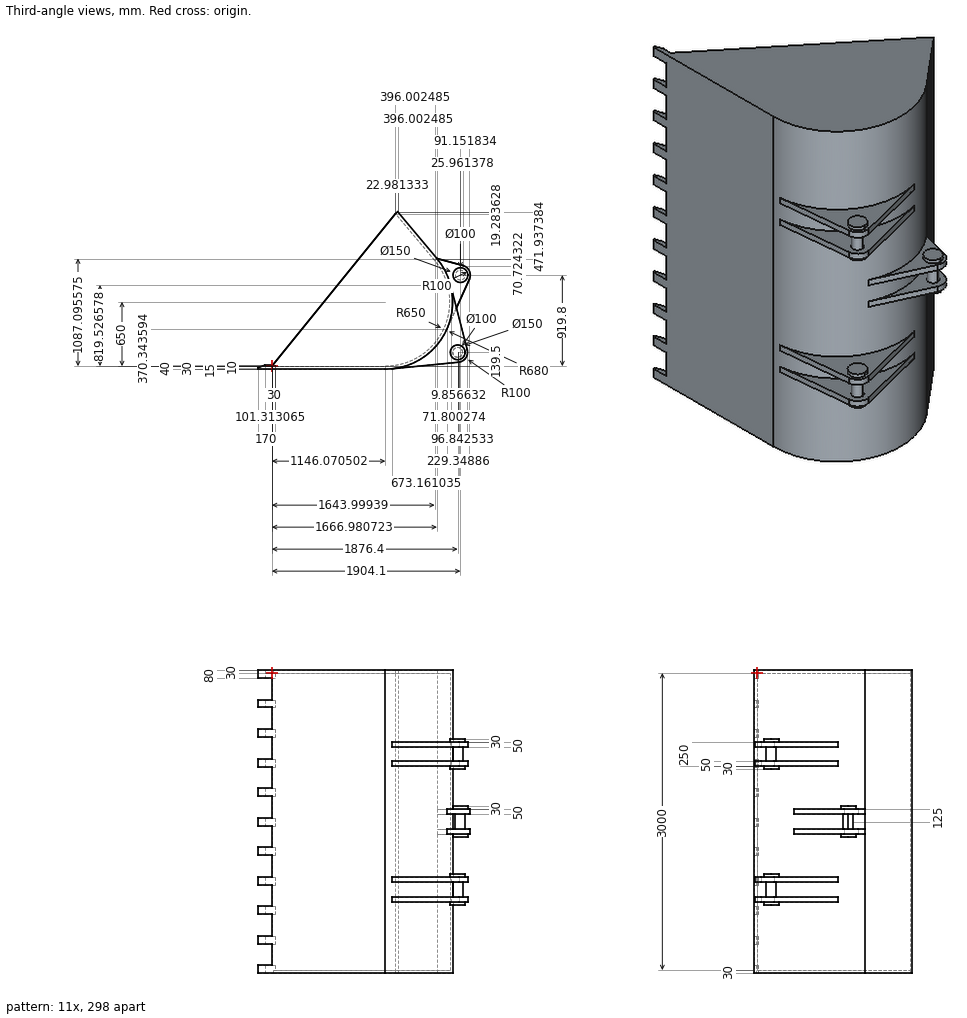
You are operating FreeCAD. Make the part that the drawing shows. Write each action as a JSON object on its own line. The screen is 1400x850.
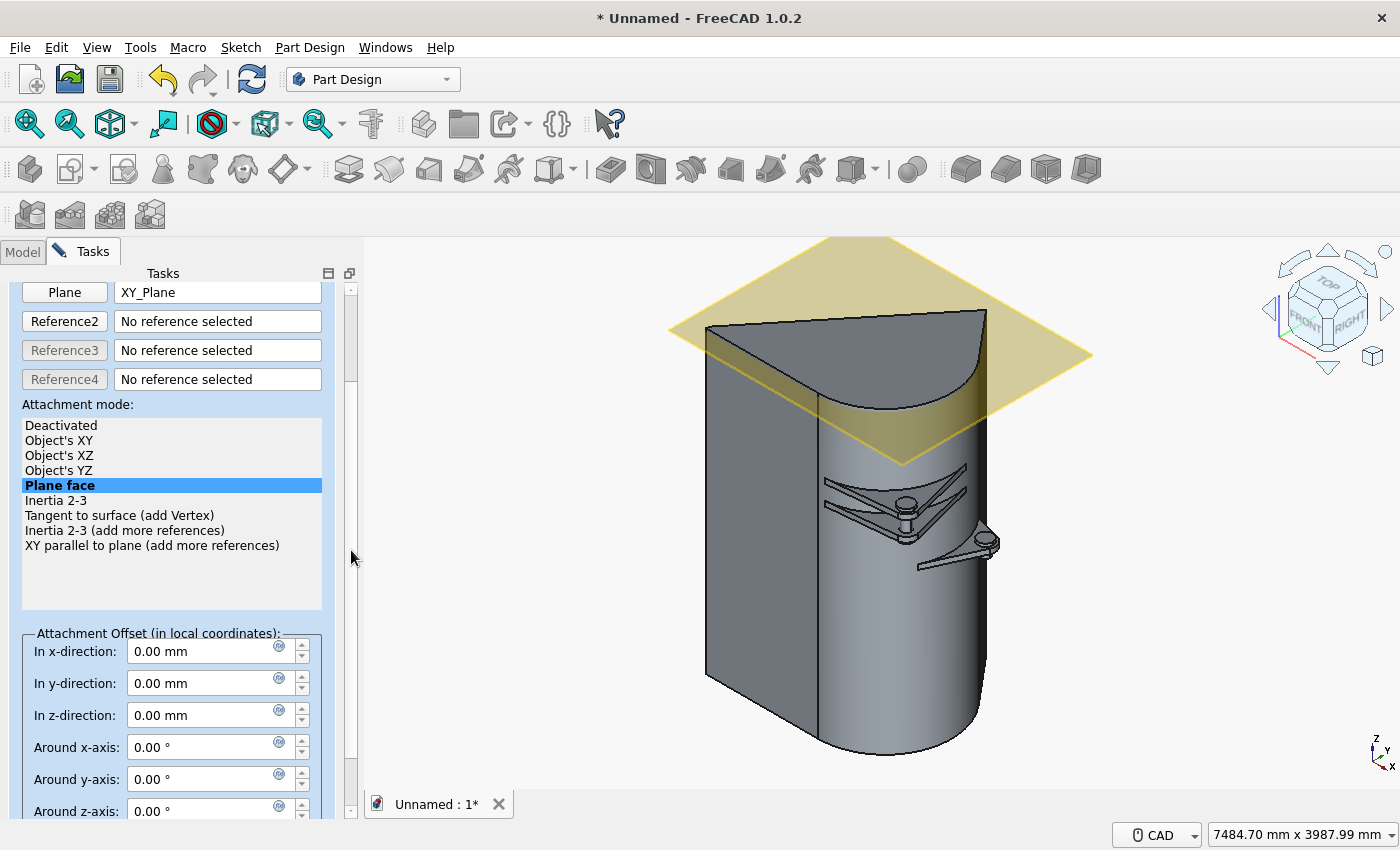
{"action": "triple_click", "coordinate": [210, 715]}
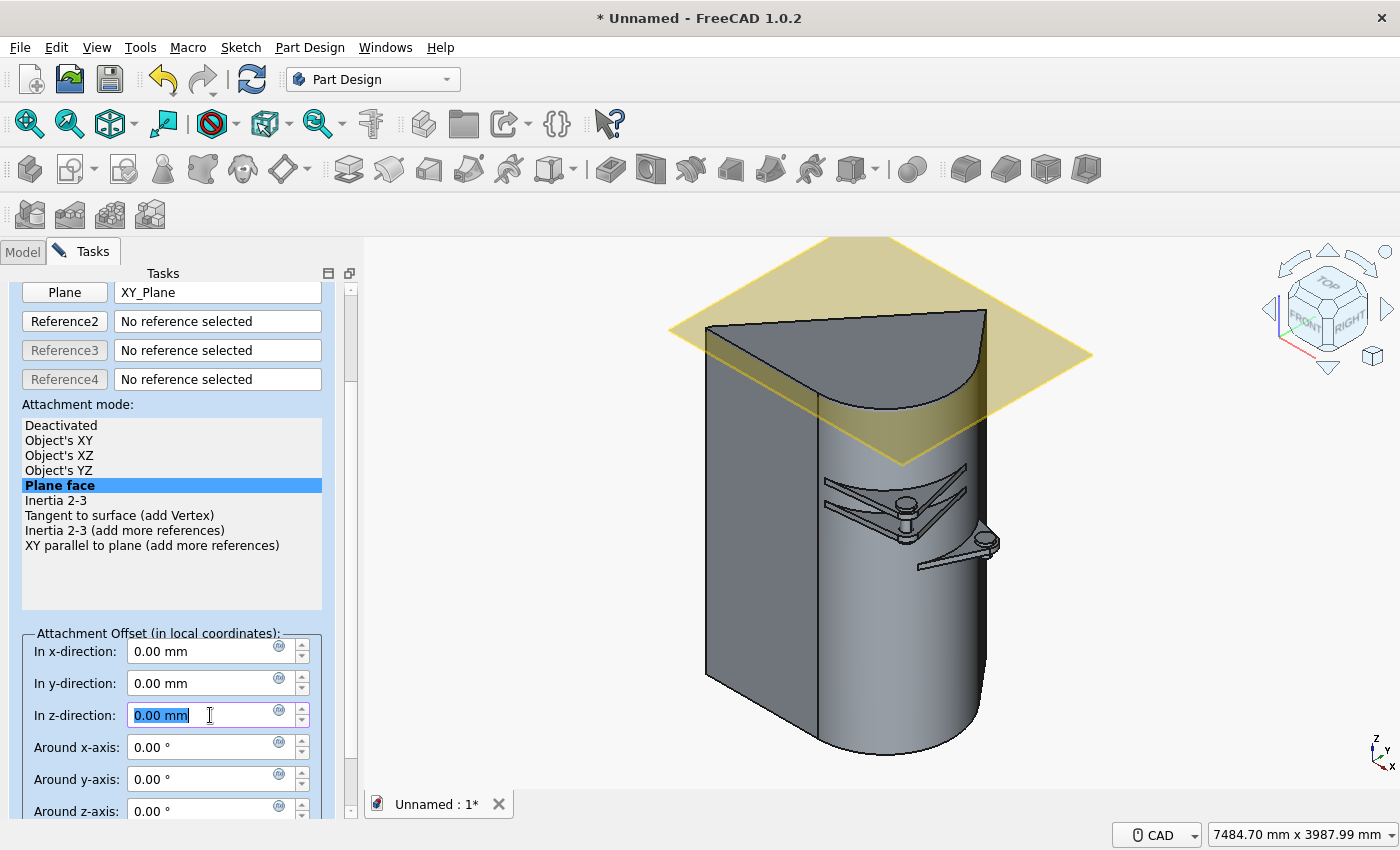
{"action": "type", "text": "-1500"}
{"action": "key", "text": "Tab"}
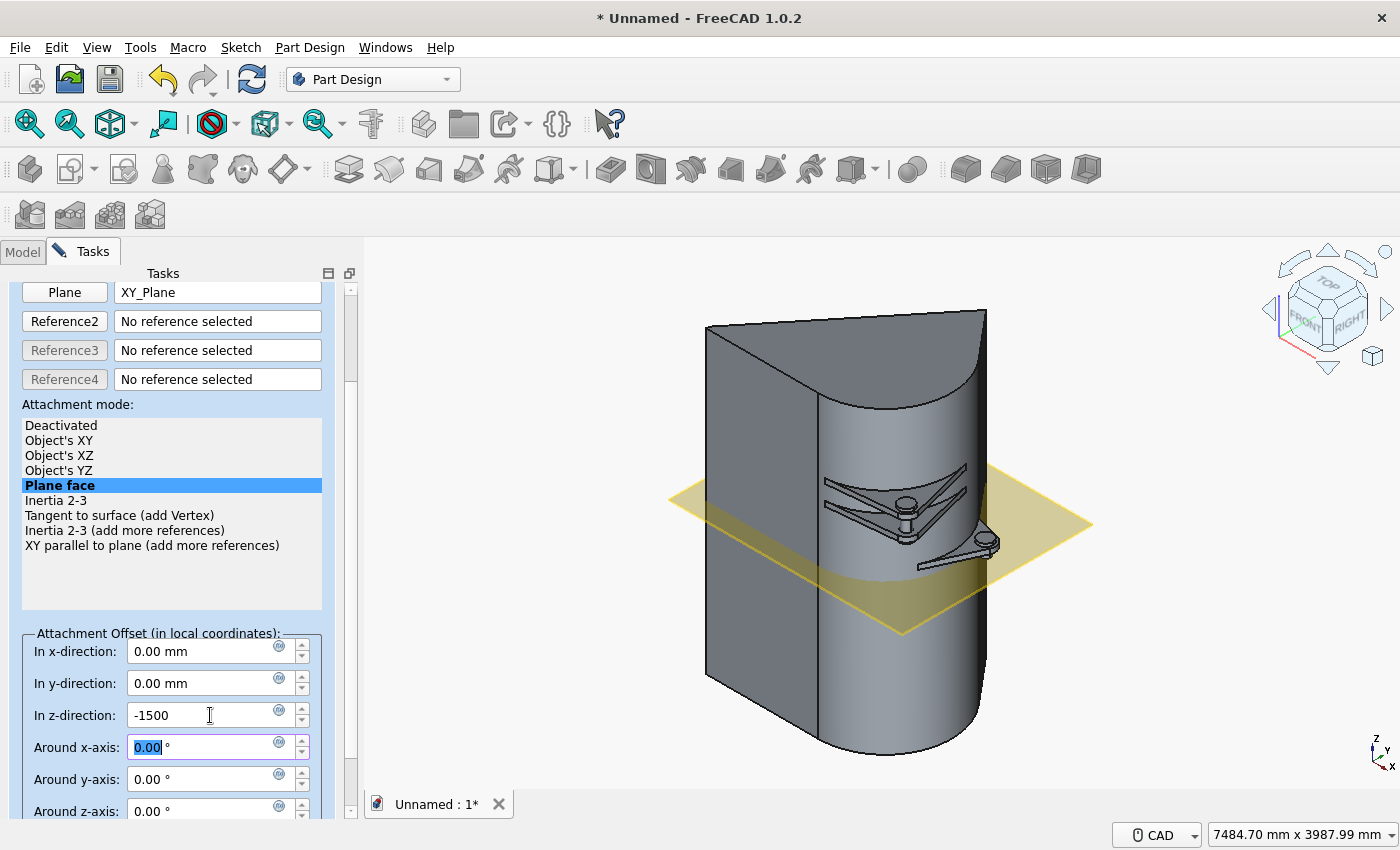
{"action": "scroll", "coordinate": [351, 550], "scroll_direction": "up", "scroll_amount": 3}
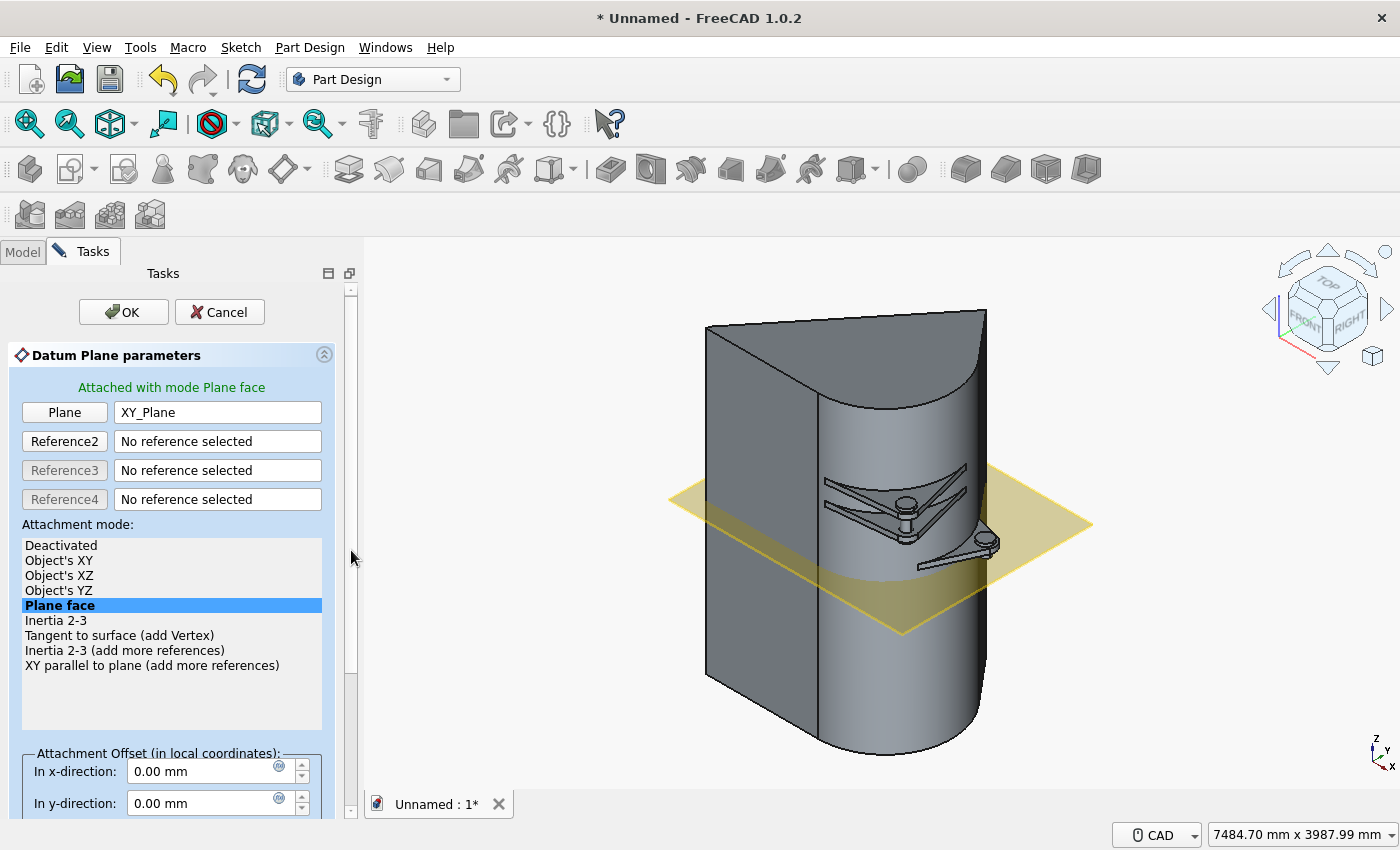
{"action": "left_click", "coordinate": [124, 312]}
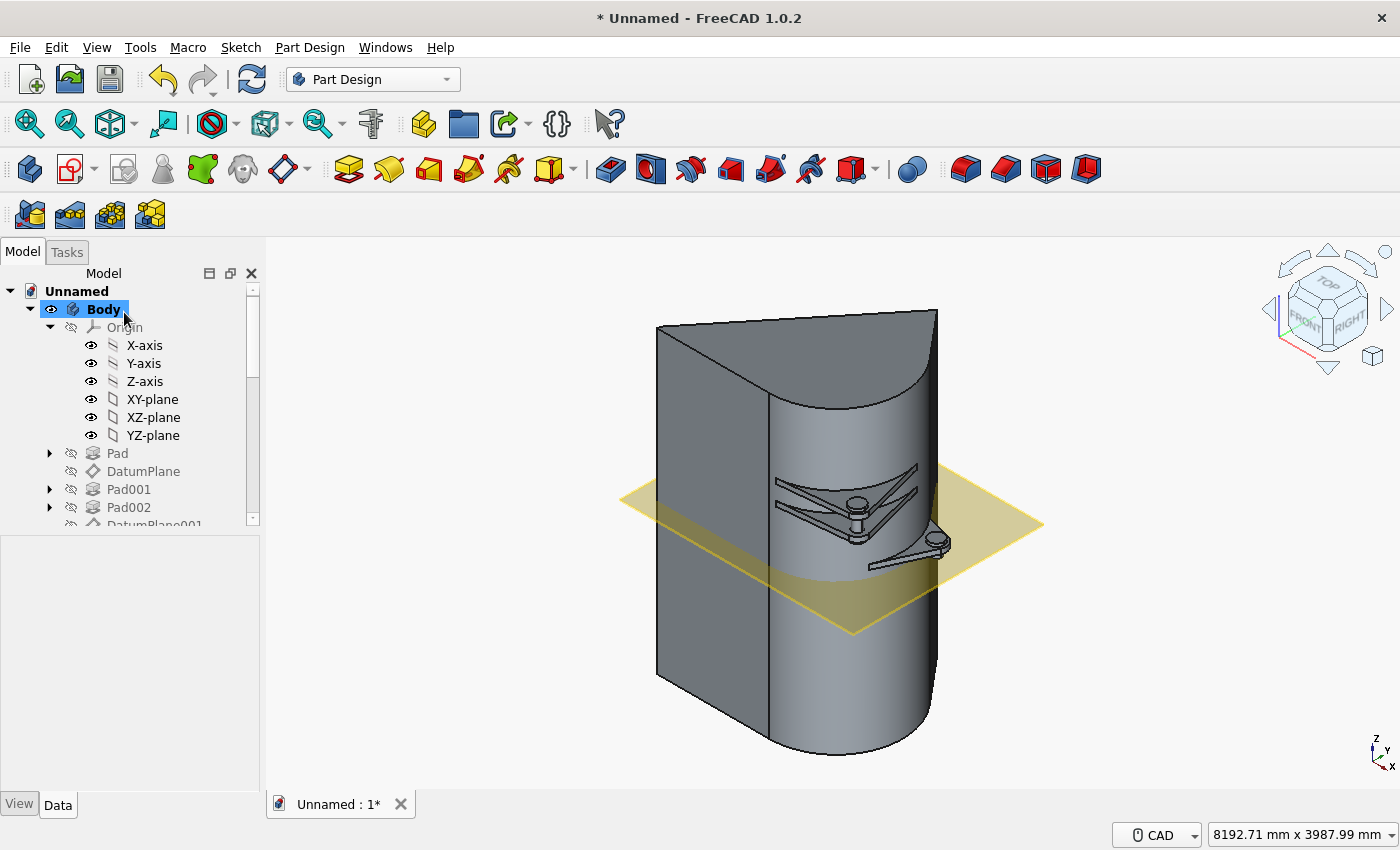
{"action": "scroll", "coordinate": [100, 413], "scroll_direction": "down", "scroll_amount": 3}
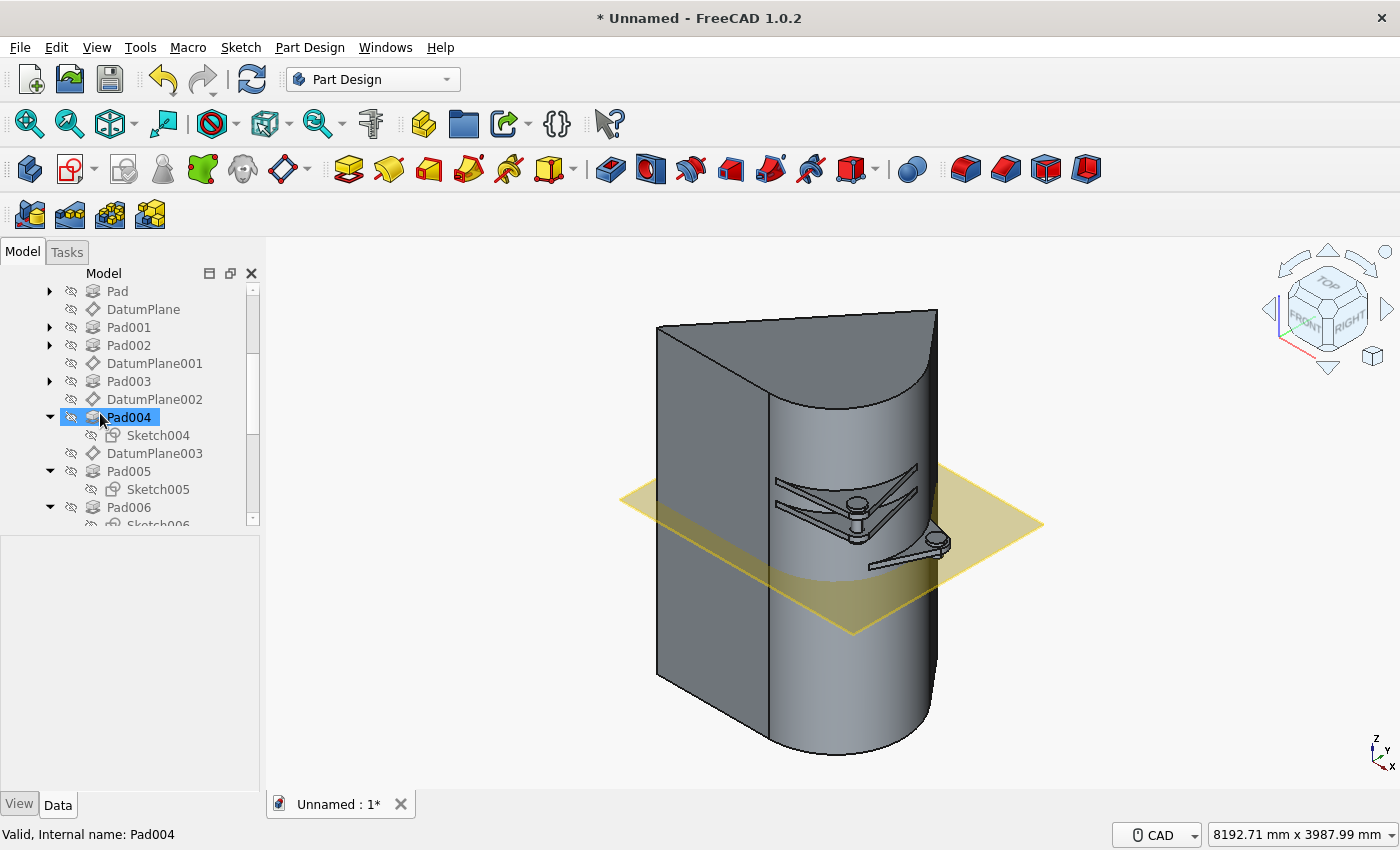
{"action": "left_click", "coordinate": [116, 381]}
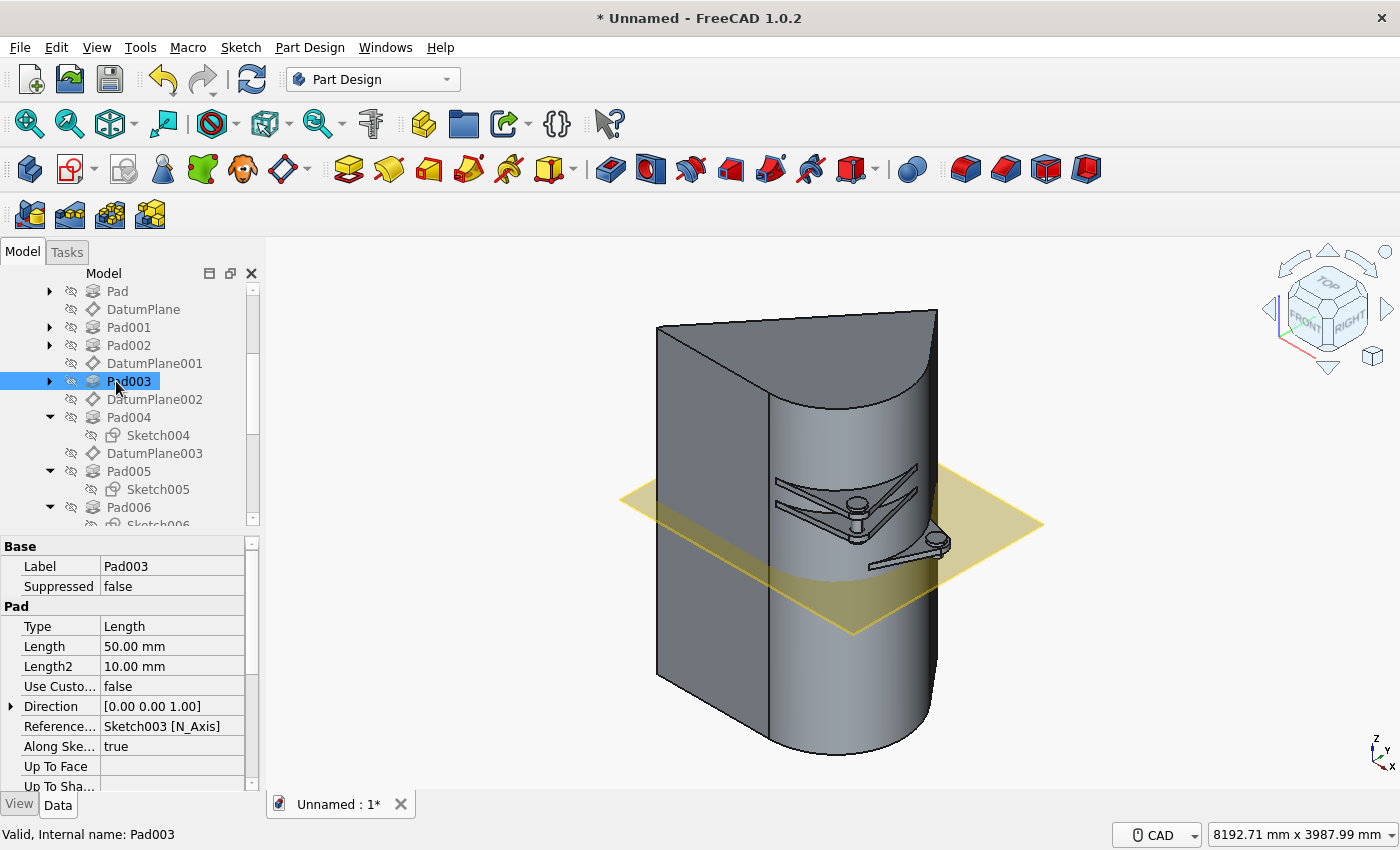
{"action": "left_click", "coordinate": [116, 417], "text": "ctrl"}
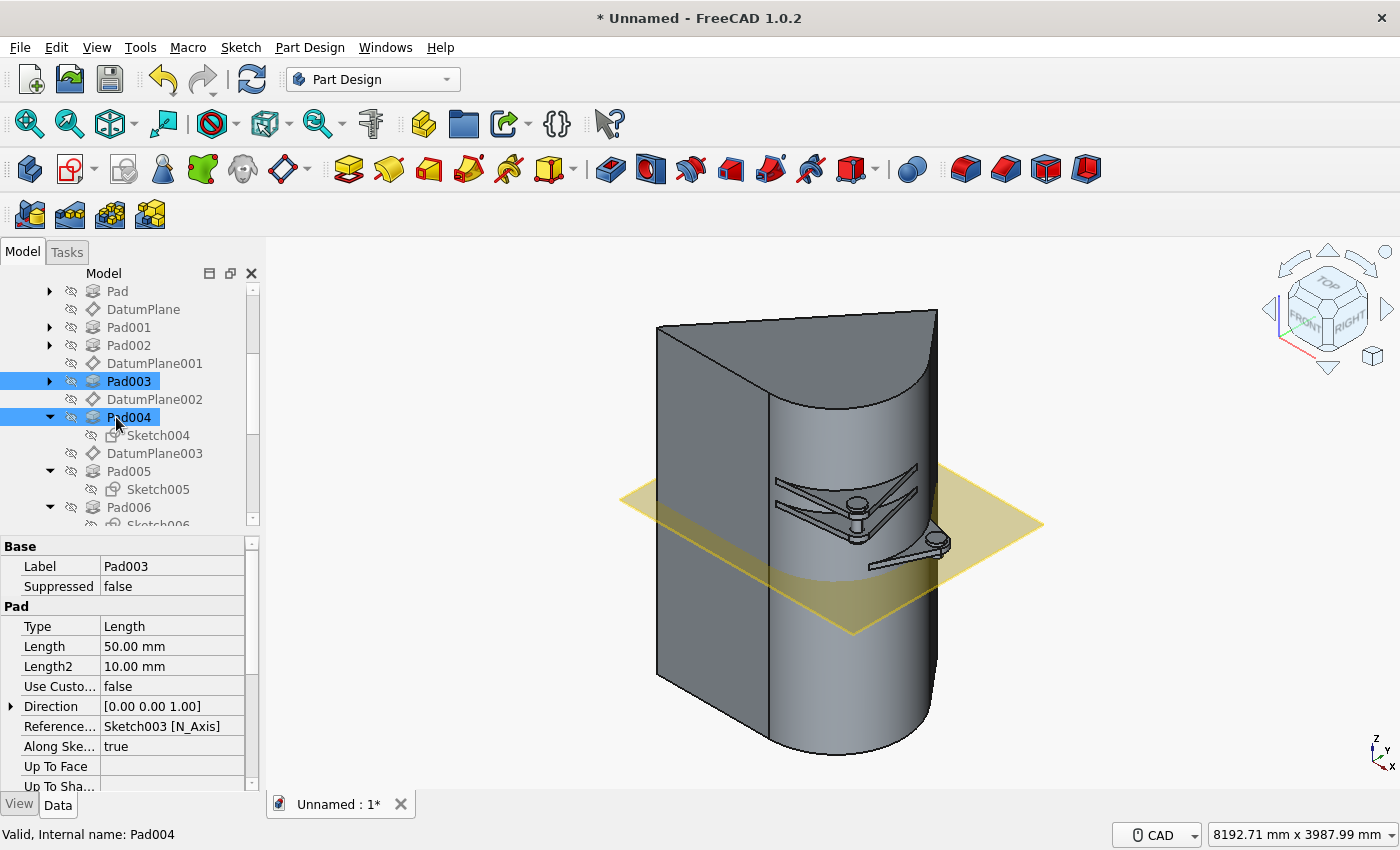
{"action": "left_click", "coordinate": [116, 471], "text": "ctrl"}